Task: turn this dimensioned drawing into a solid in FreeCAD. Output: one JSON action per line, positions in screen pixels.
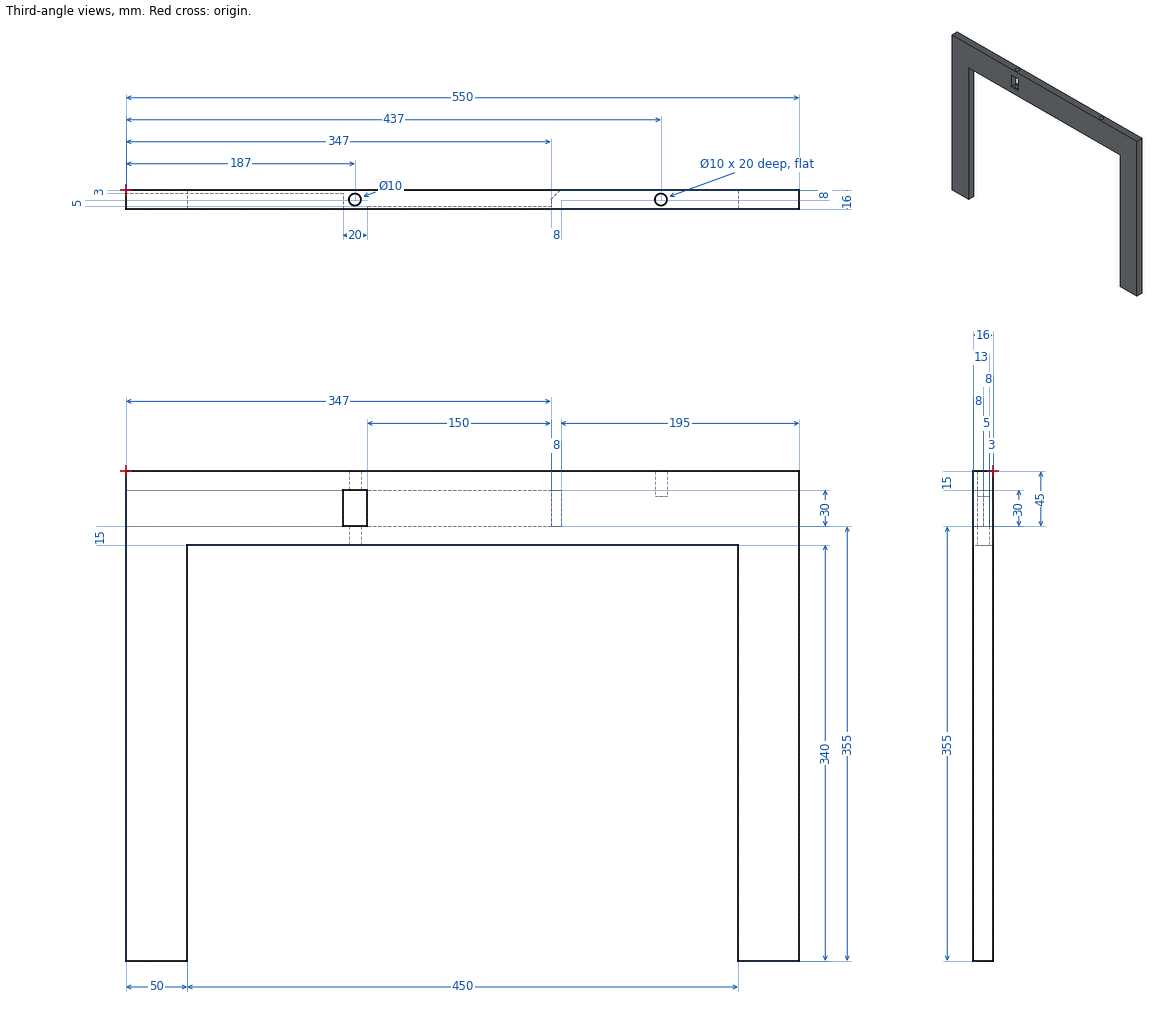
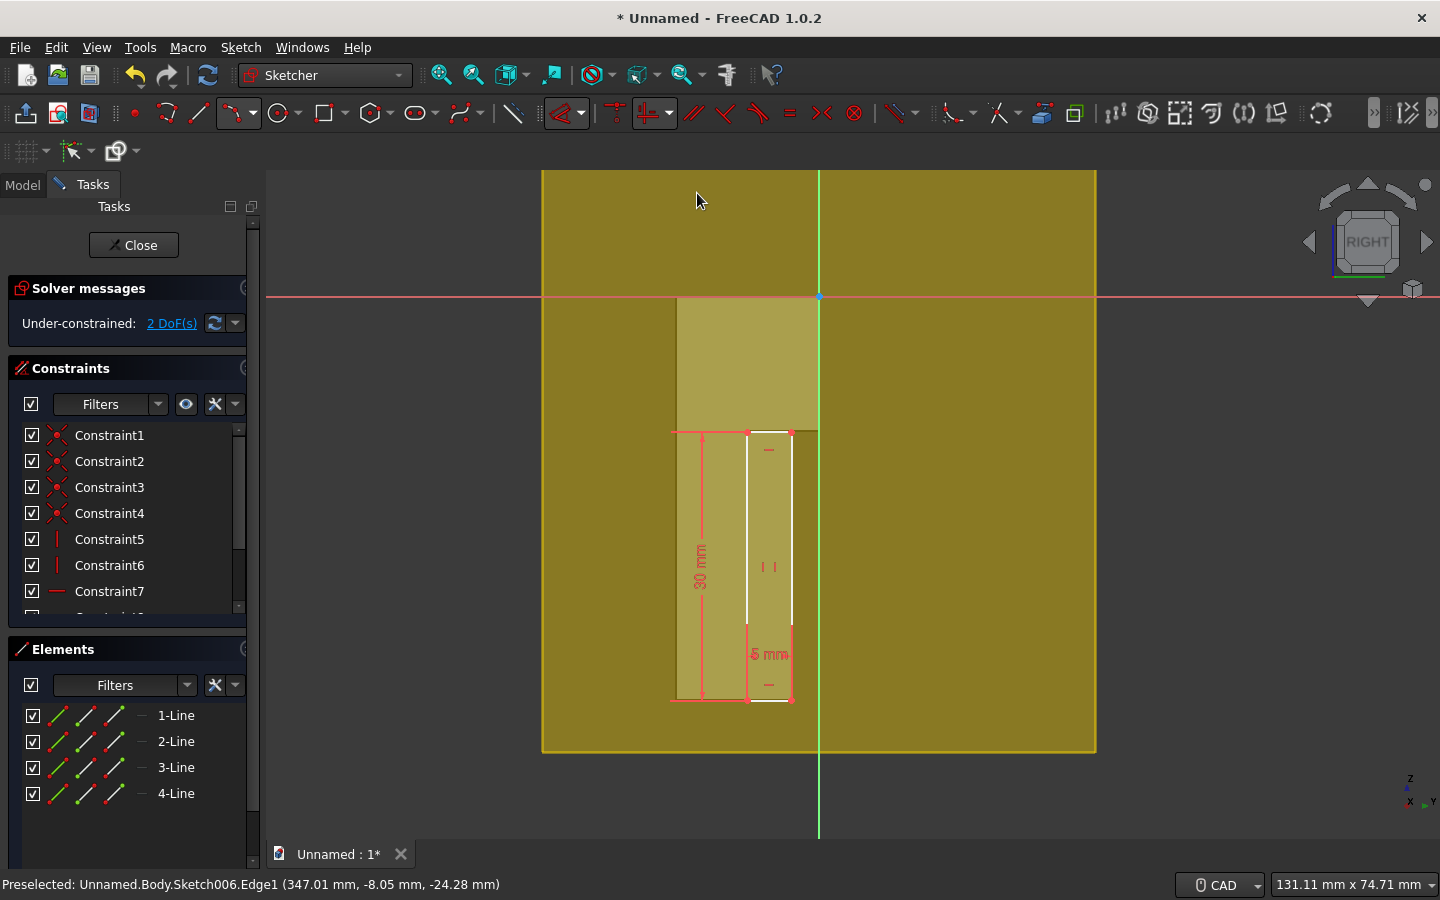
{"action": "left_click", "coordinate": [747, 432]}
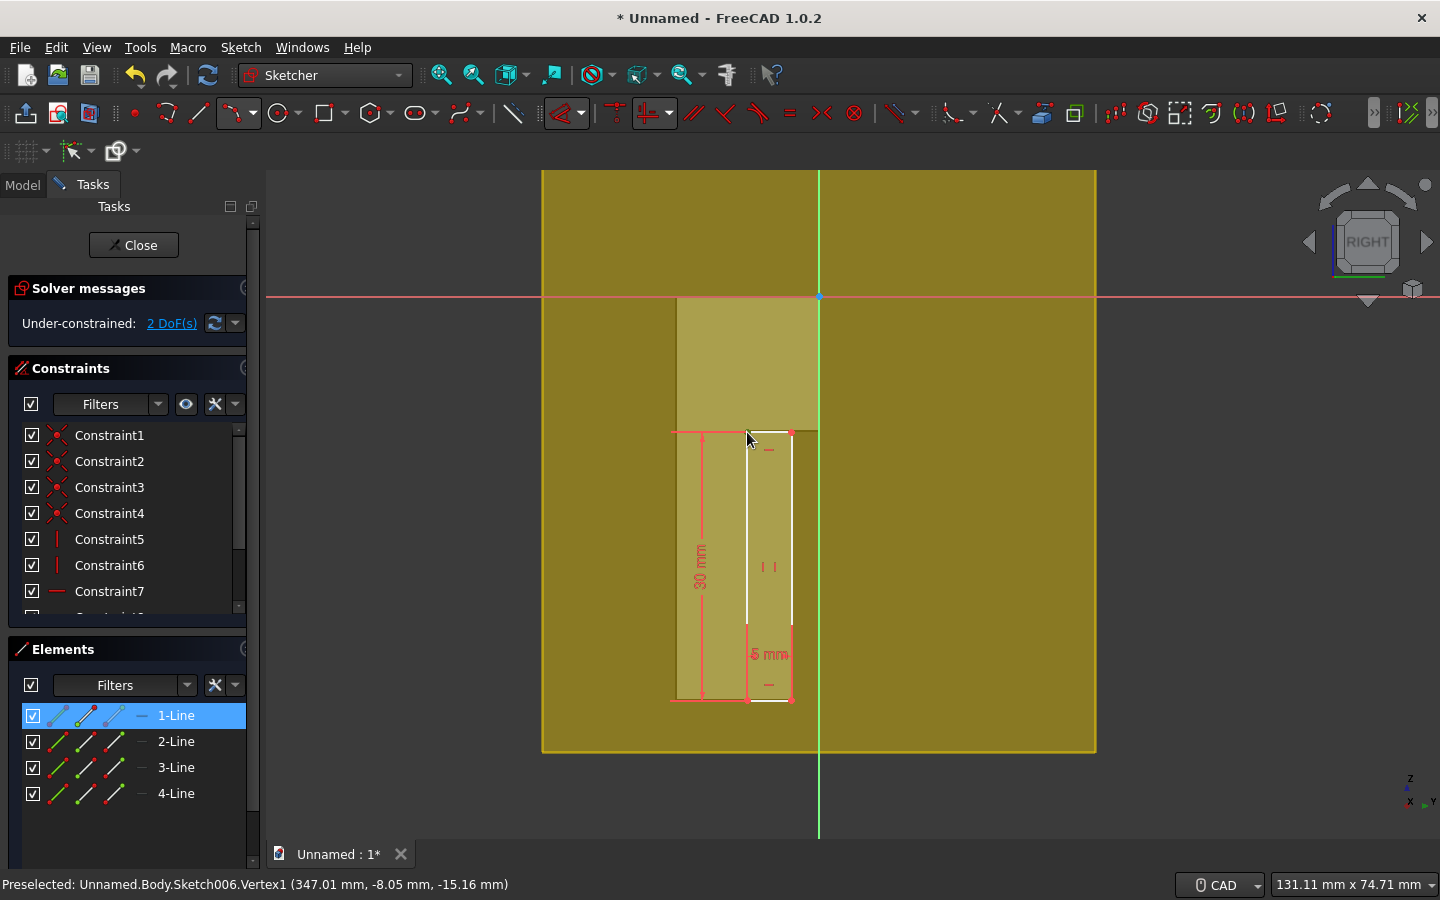
{"action": "left_click", "coordinate": [584, 114]}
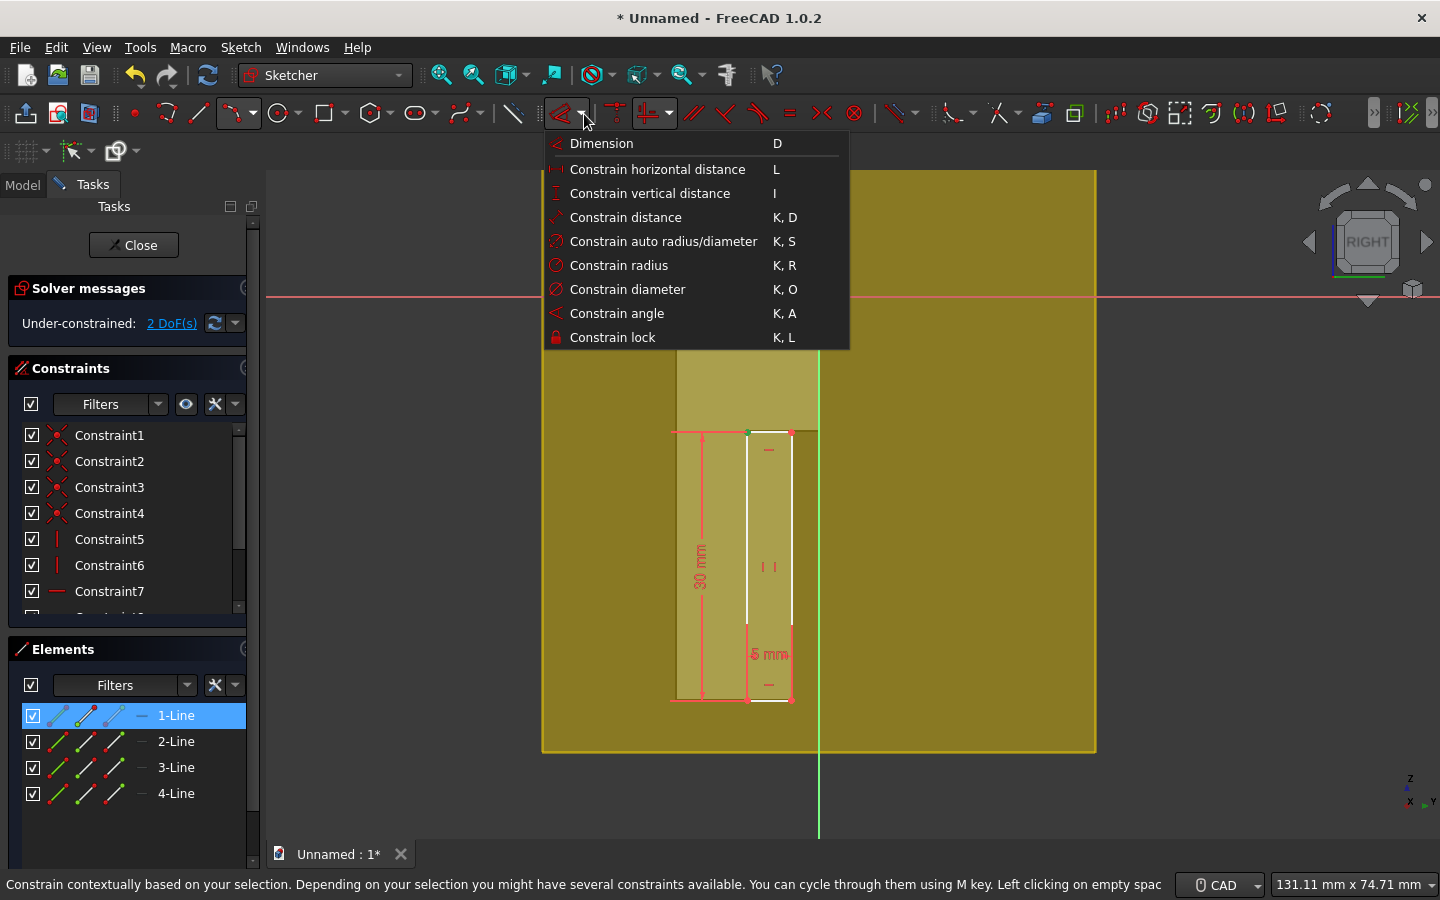
{"action": "left_click", "coordinate": [697, 169]}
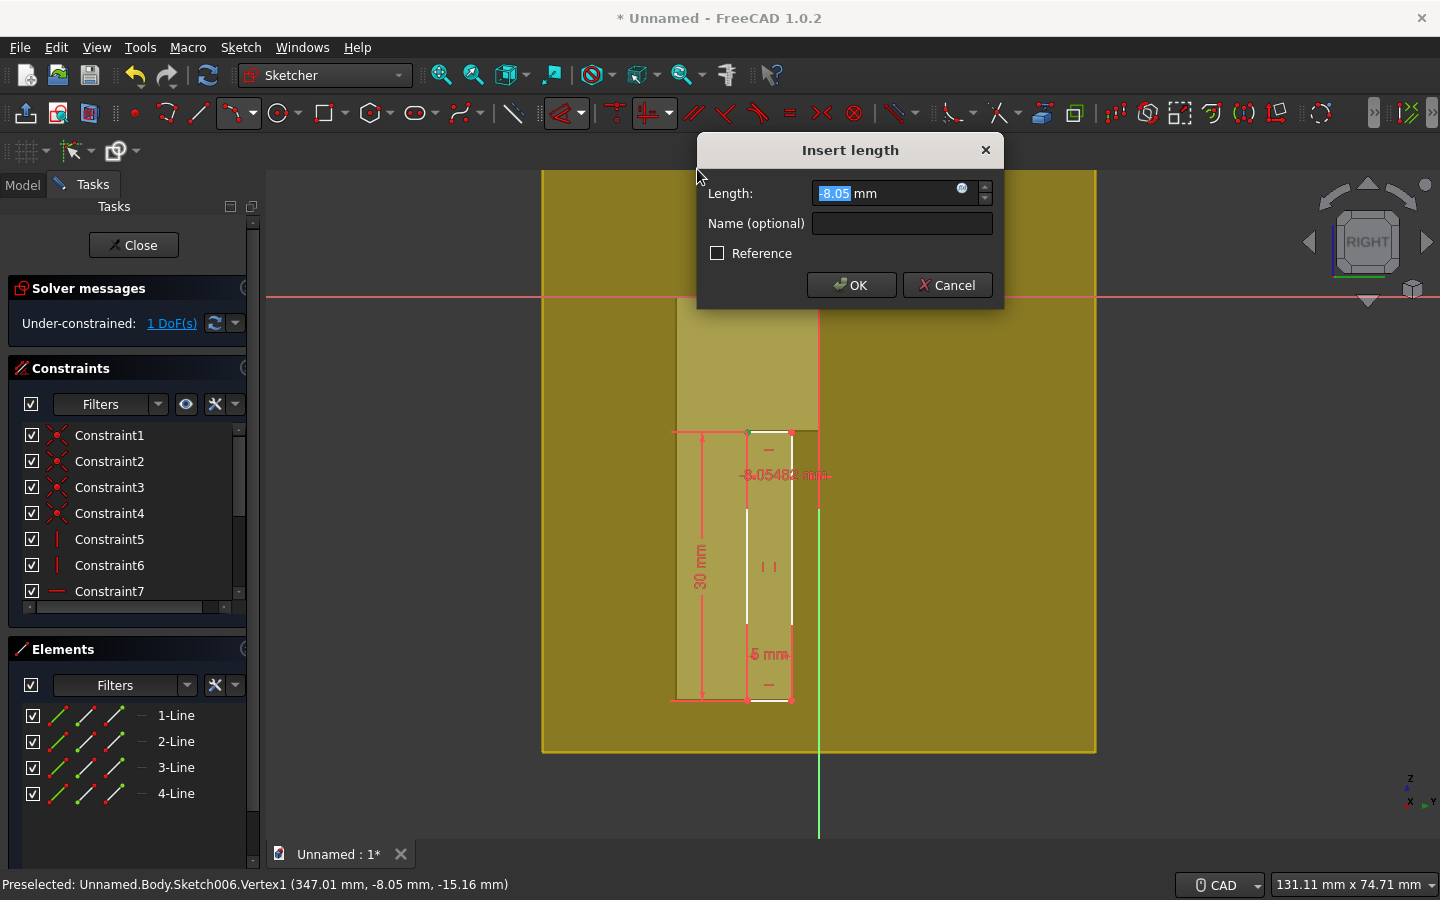
{"action": "type", "text": "-8"}
{"action": "key", "text": "Return"}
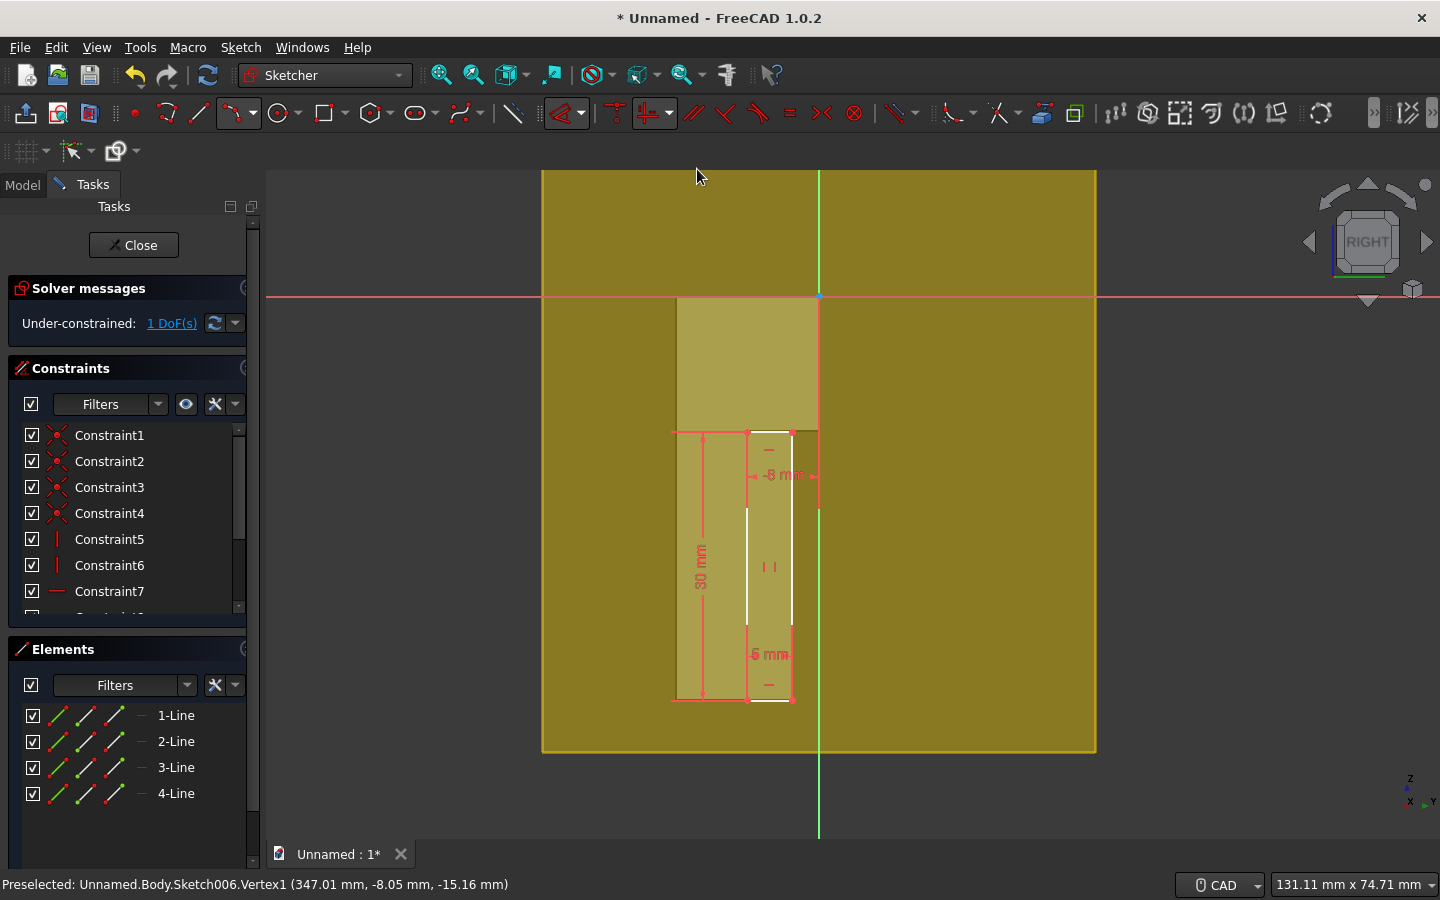
{"action": "left_click", "coordinate": [747, 432]}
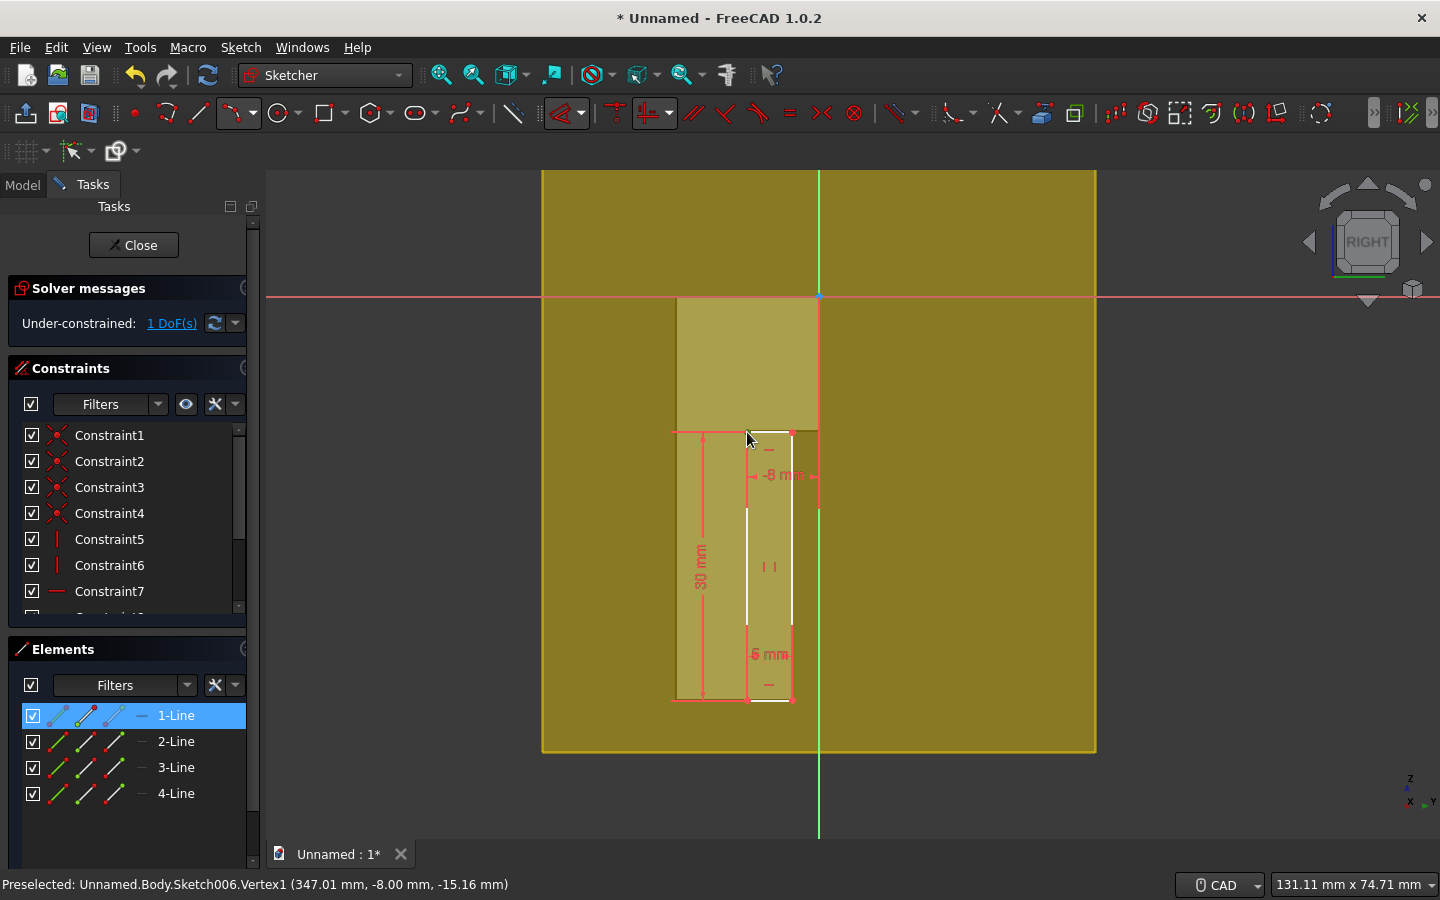
{"action": "left_click", "coordinate": [584, 114]}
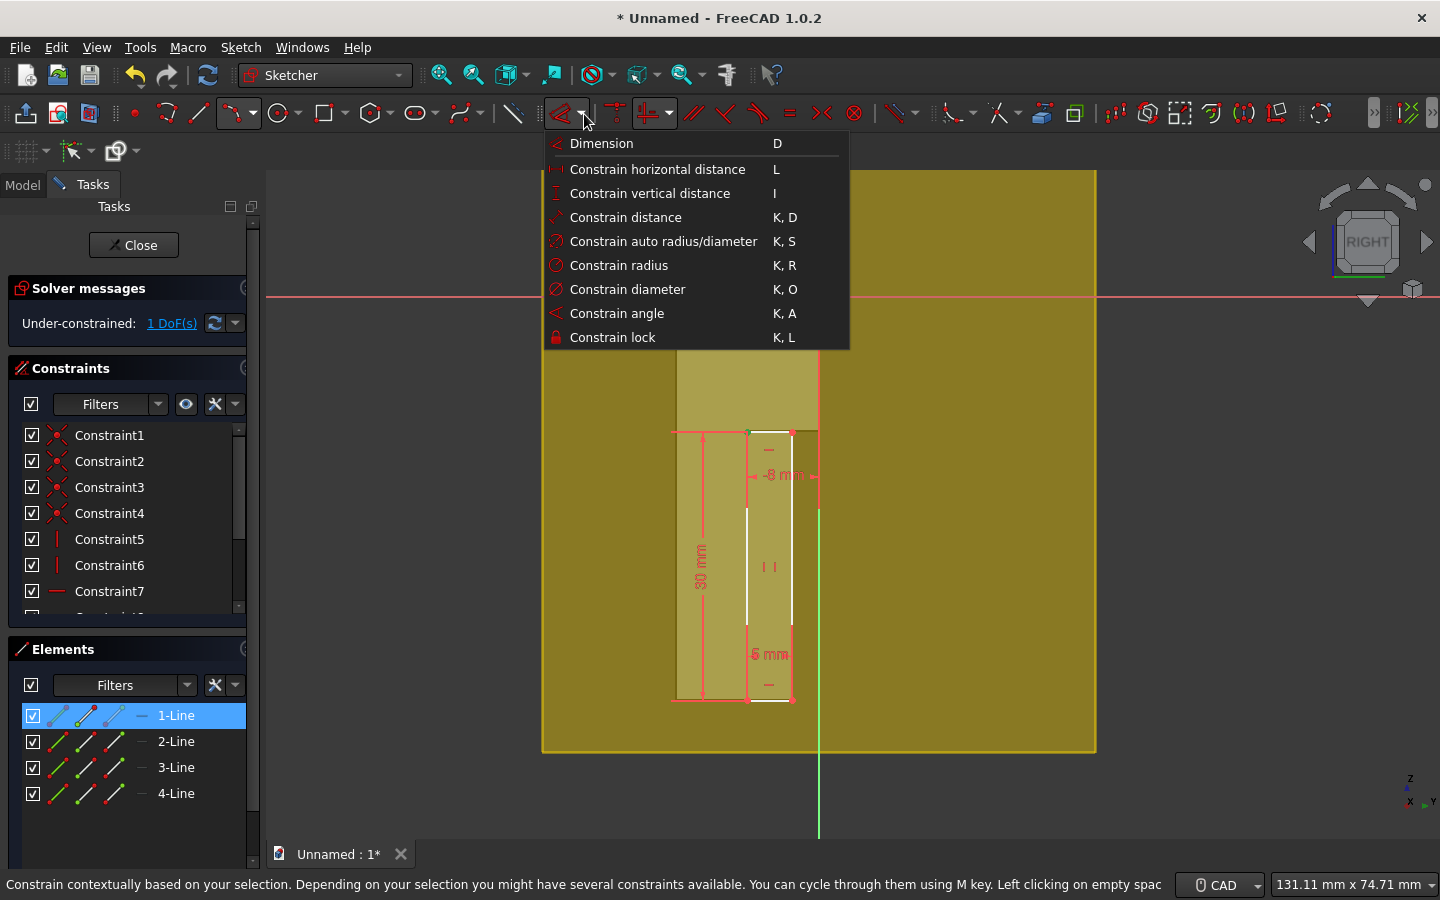
{"action": "left_click", "coordinate": [697, 193]}